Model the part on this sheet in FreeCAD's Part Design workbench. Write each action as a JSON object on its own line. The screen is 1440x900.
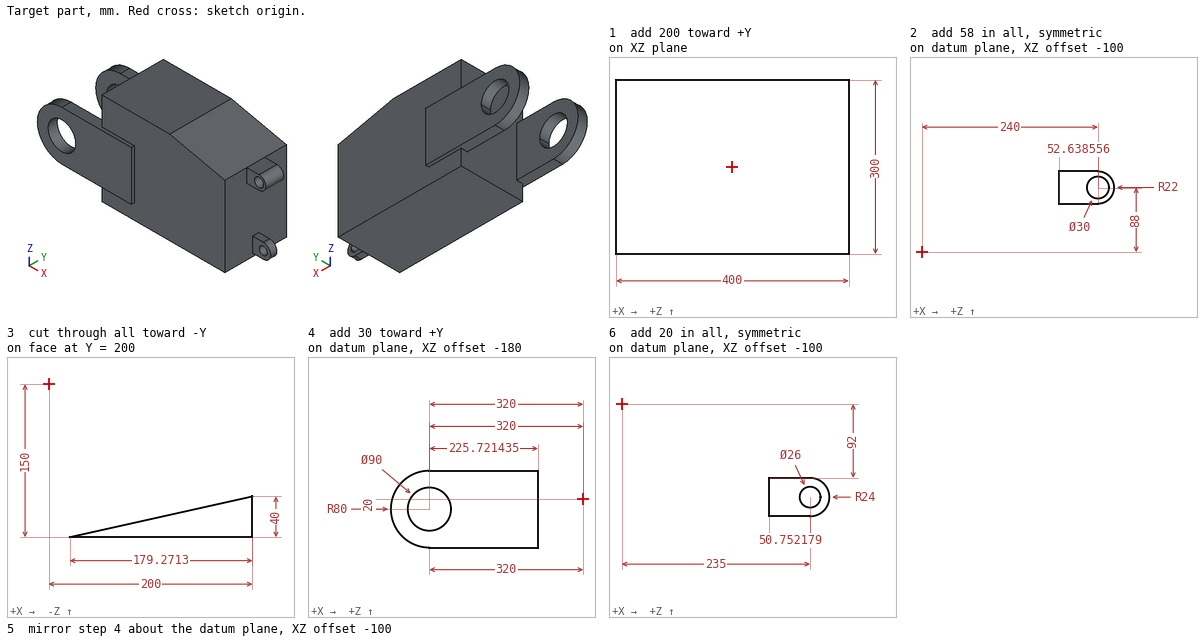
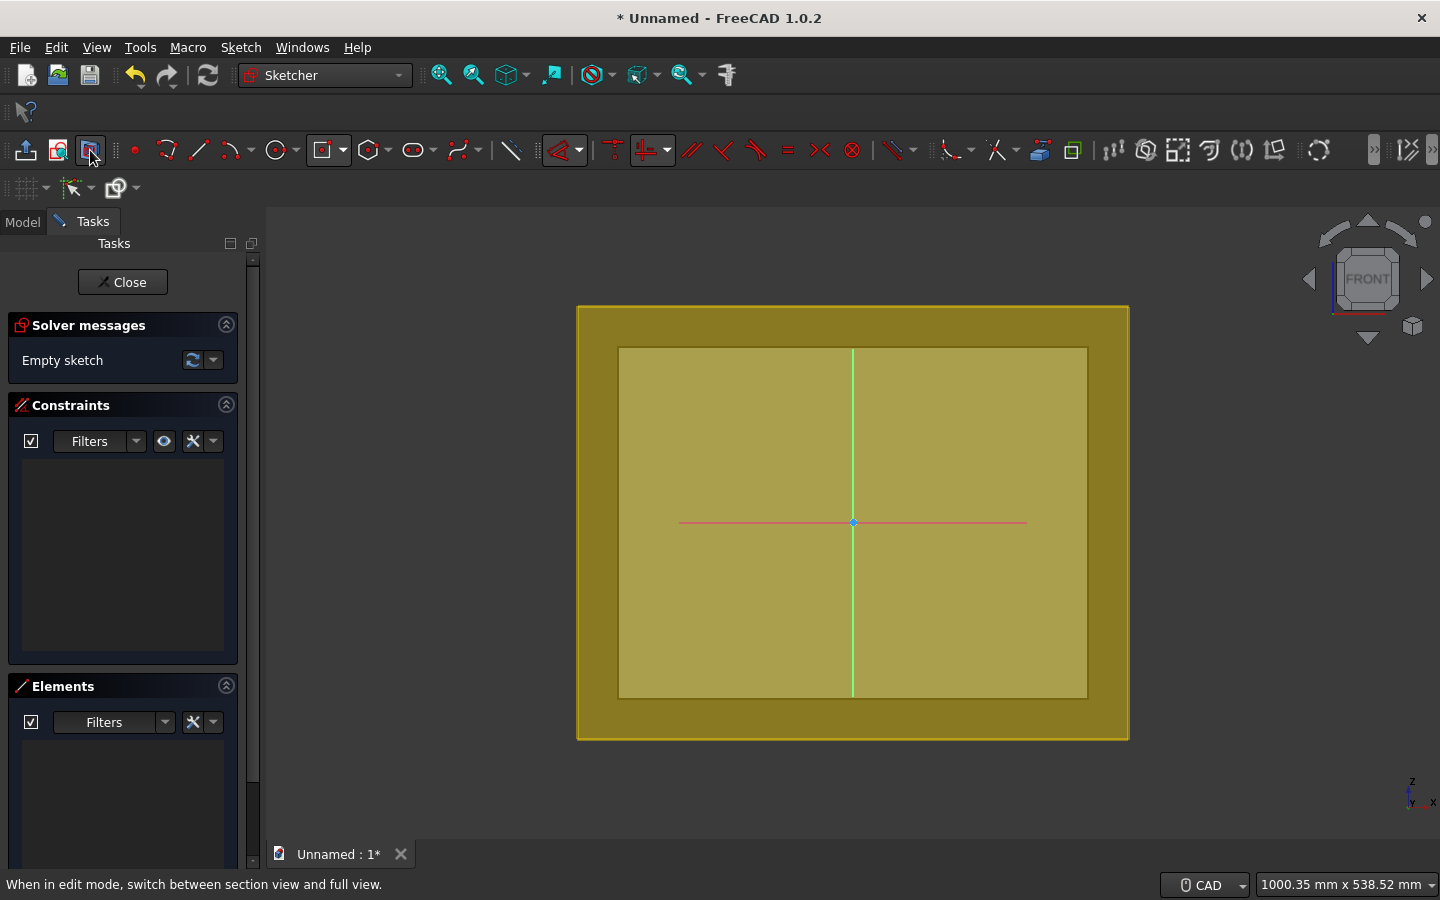
{"action": "scroll", "coordinate": [1169, 404], "scroll_direction": "up", "scroll_amount": 10}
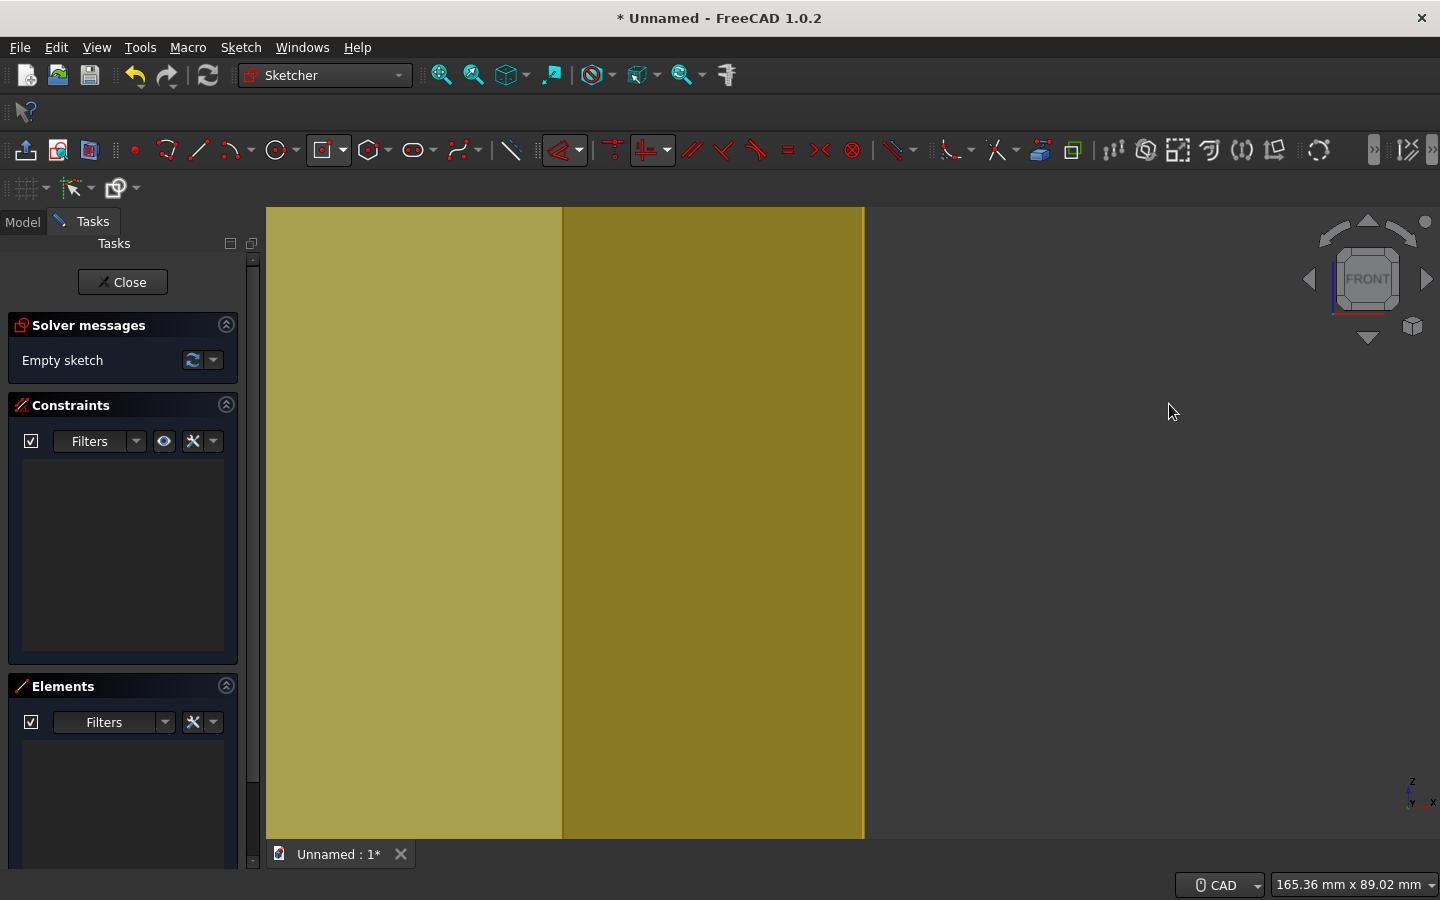
{"action": "left_click", "coordinate": [168, 150]}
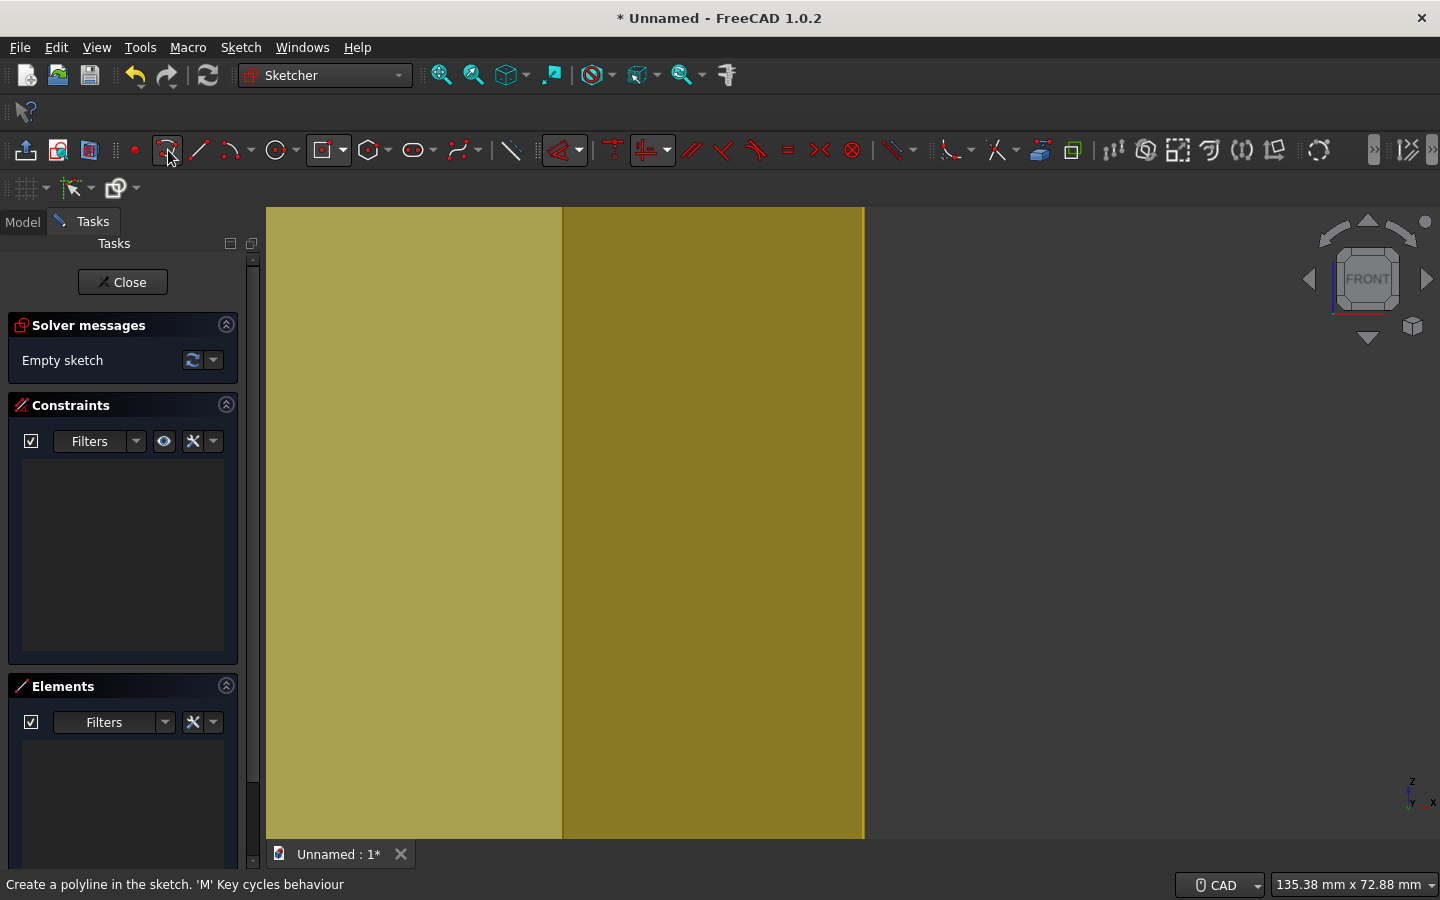
{"action": "left_click", "coordinate": [910, 709]}
{"action": "left_click", "coordinate": [454, 709]}
{"action": "left_click", "coordinate": [454, 327]}
{"action": "left_click", "coordinate": [910, 327]}
{"action": "right_click", "coordinate": [910, 327]}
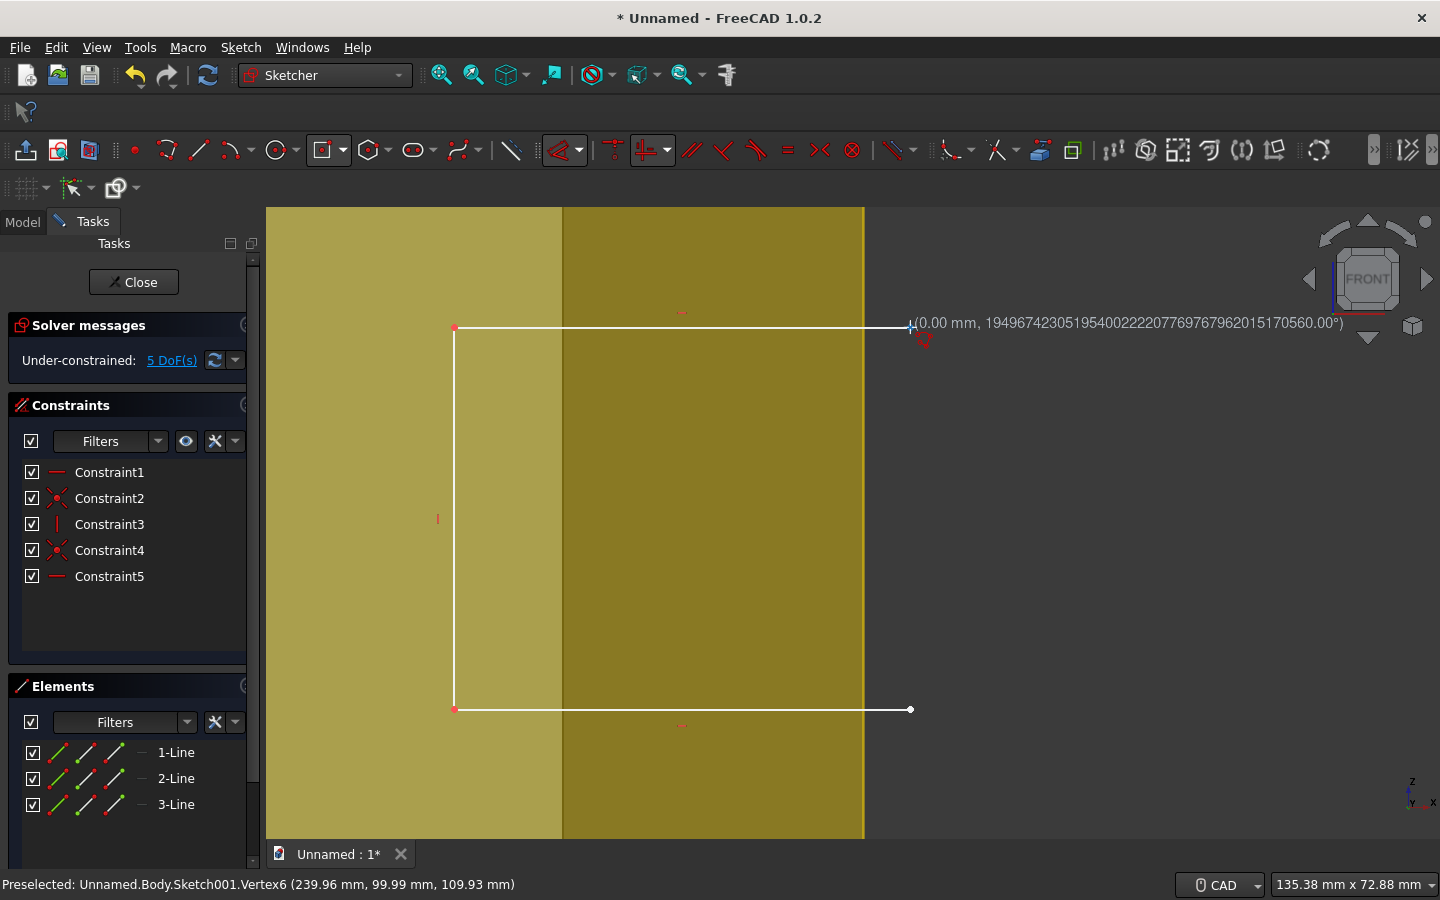
{"action": "left_click", "coordinate": [254, 150]}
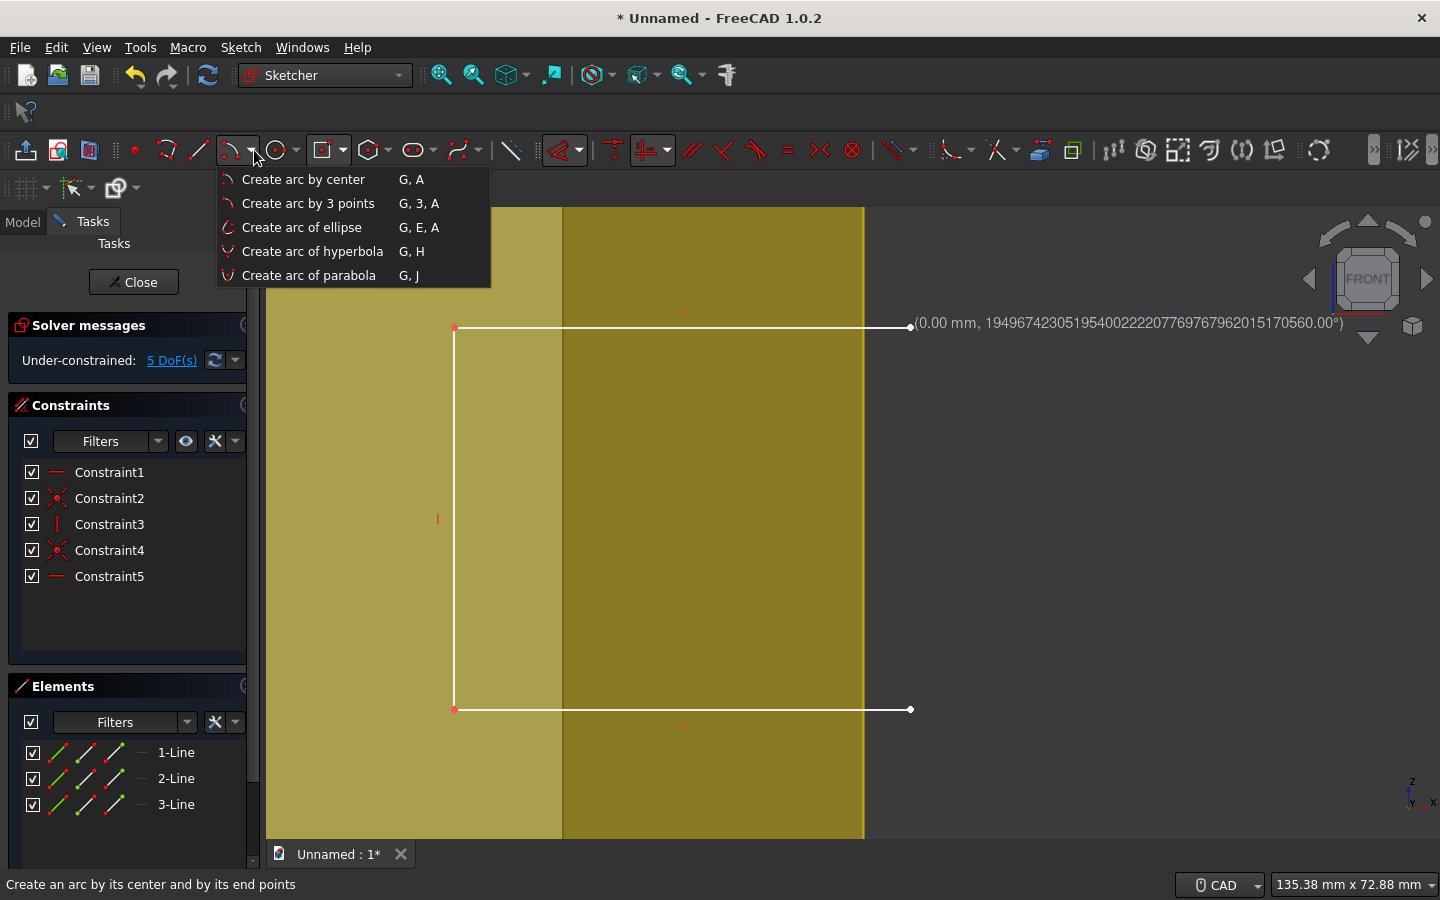
{"action": "left_click", "coordinate": [354, 203]}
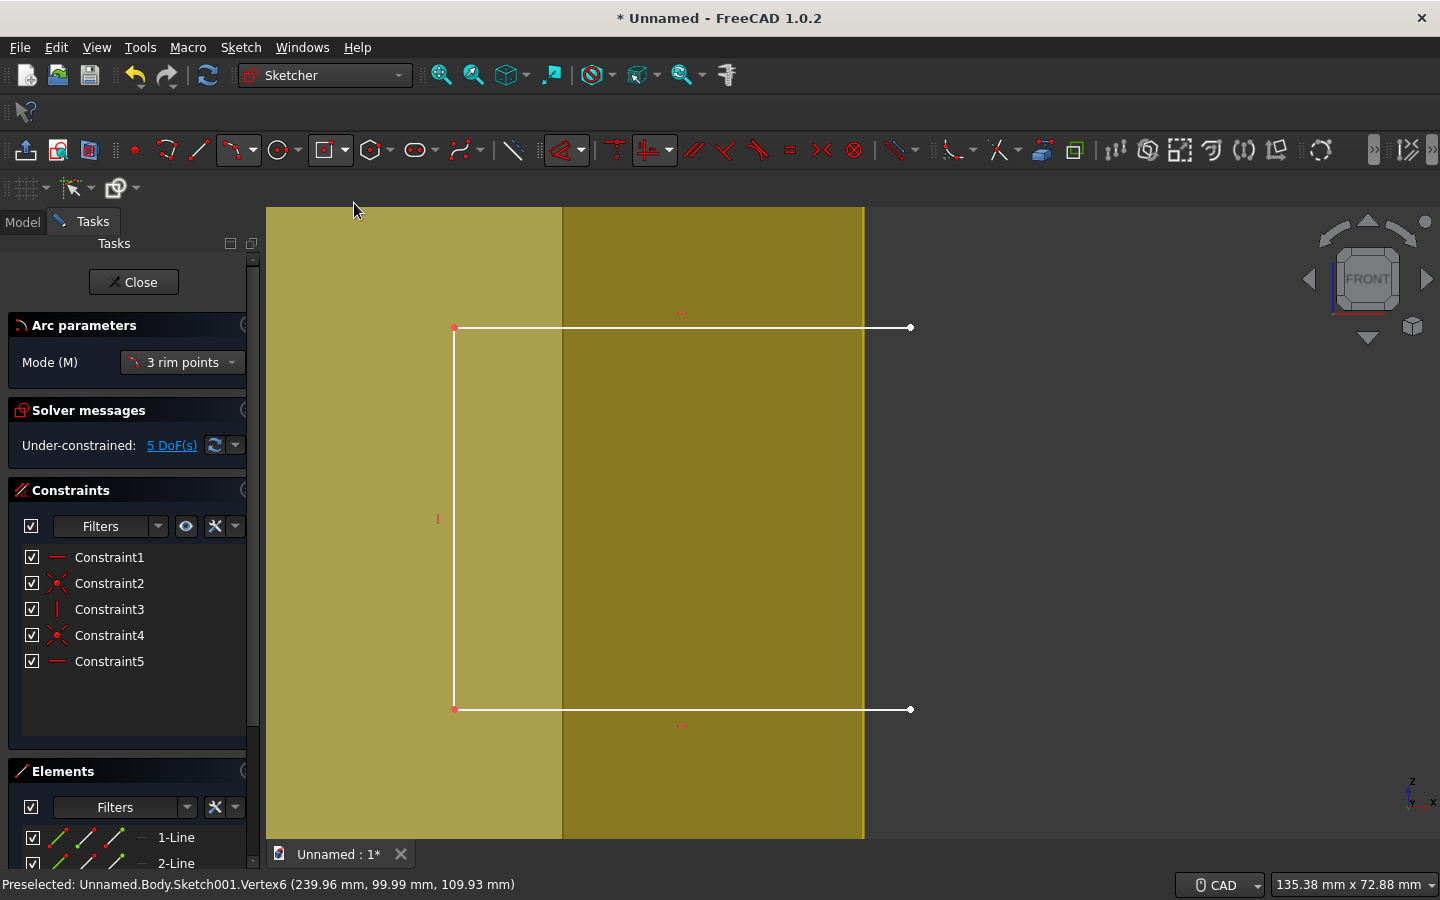
{"action": "left_click", "coordinate": [910, 328]}
{"action": "left_click", "coordinate": [910, 710]}
{"action": "left_click", "coordinate": [1101, 518]}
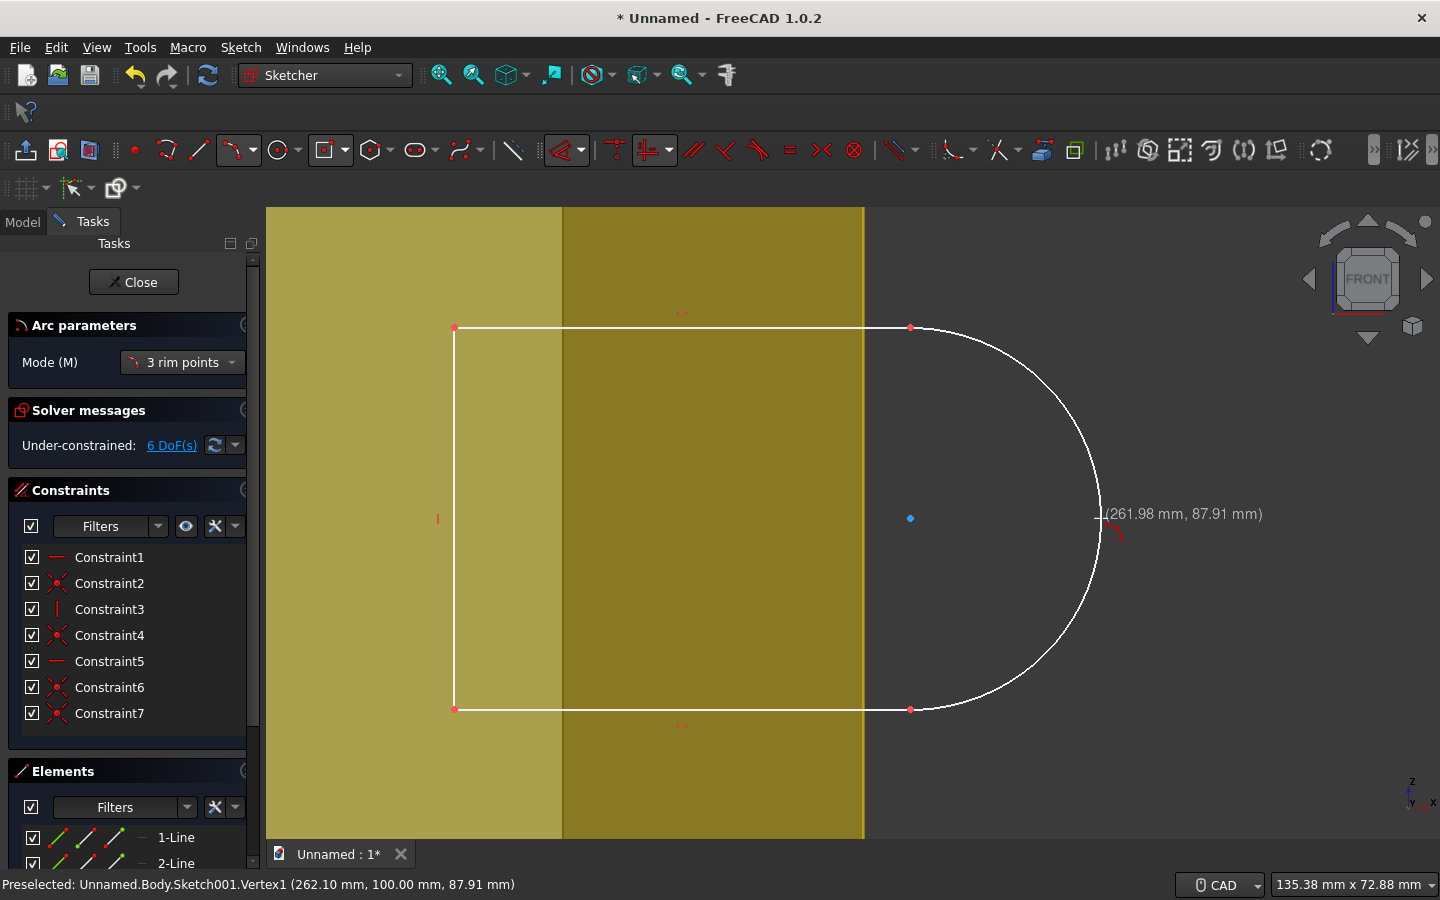
{"action": "left_click", "coordinate": [278, 150]}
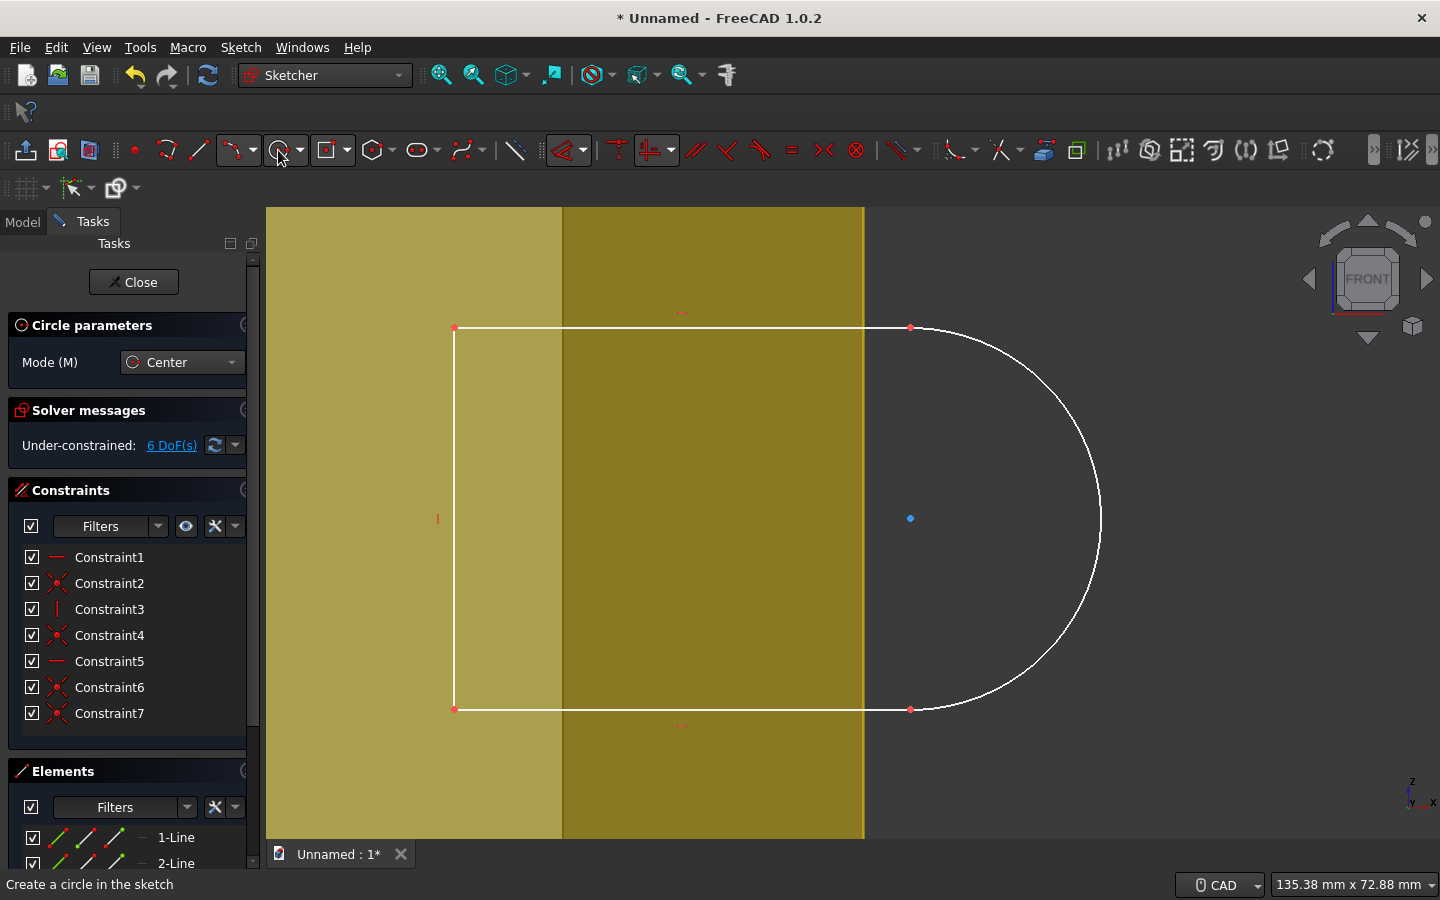
{"action": "left_click", "coordinate": [910, 518]}
{"action": "left_click", "coordinate": [1002, 426]}
{"action": "key", "text": "Escape"}